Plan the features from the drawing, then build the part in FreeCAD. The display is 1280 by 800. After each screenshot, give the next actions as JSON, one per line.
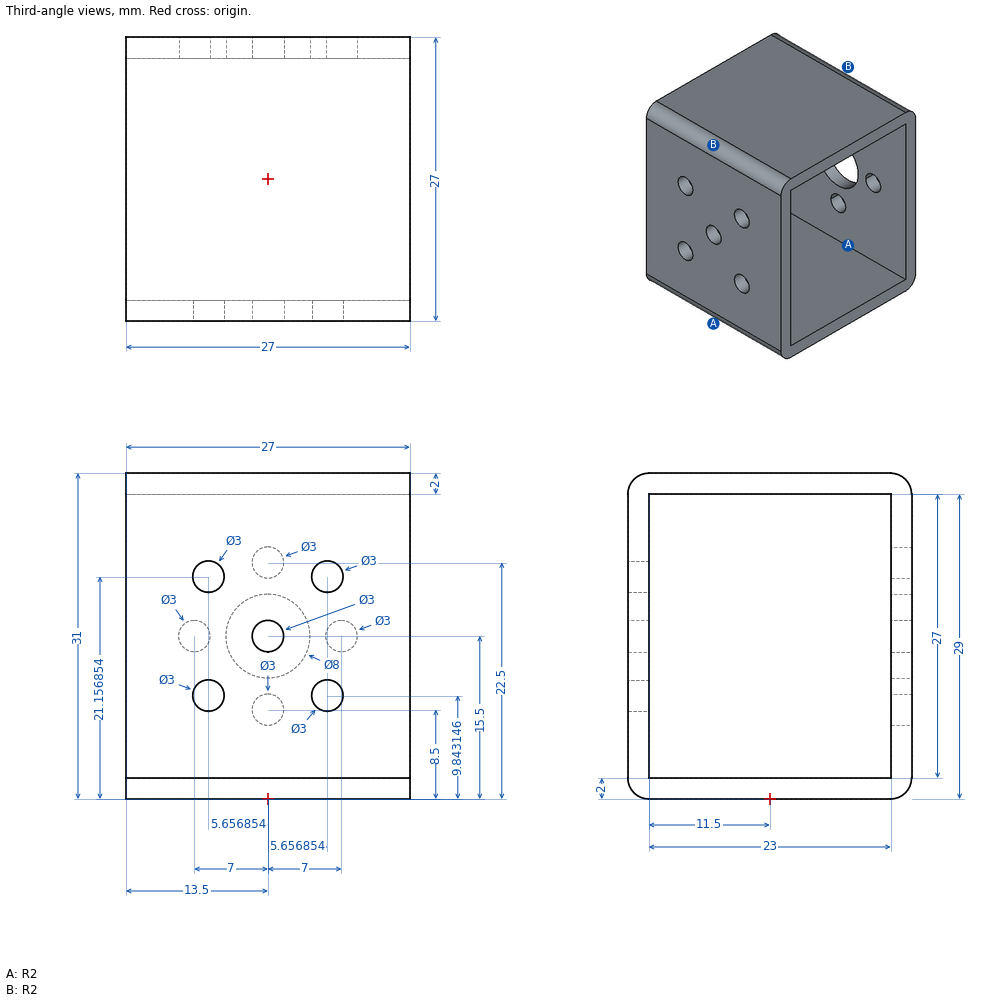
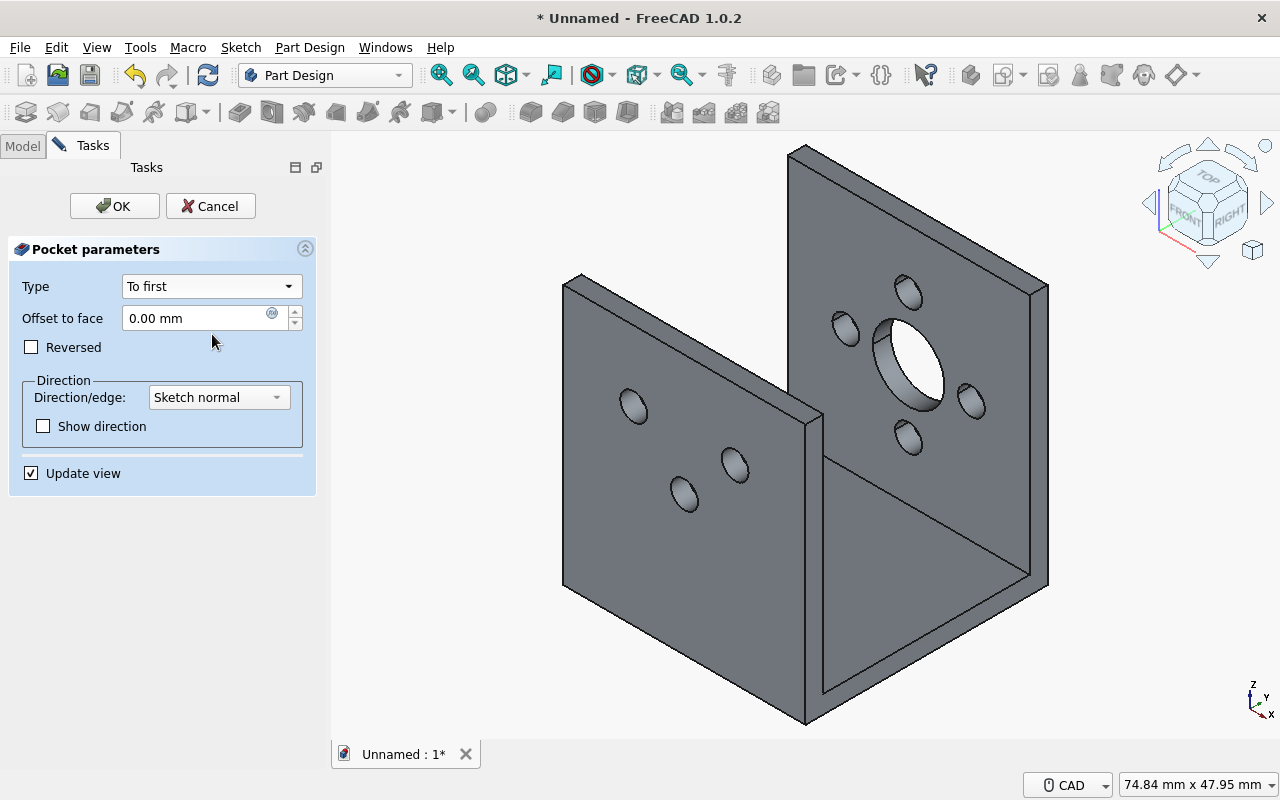
{"action": "left_click", "coordinate": [115, 206]}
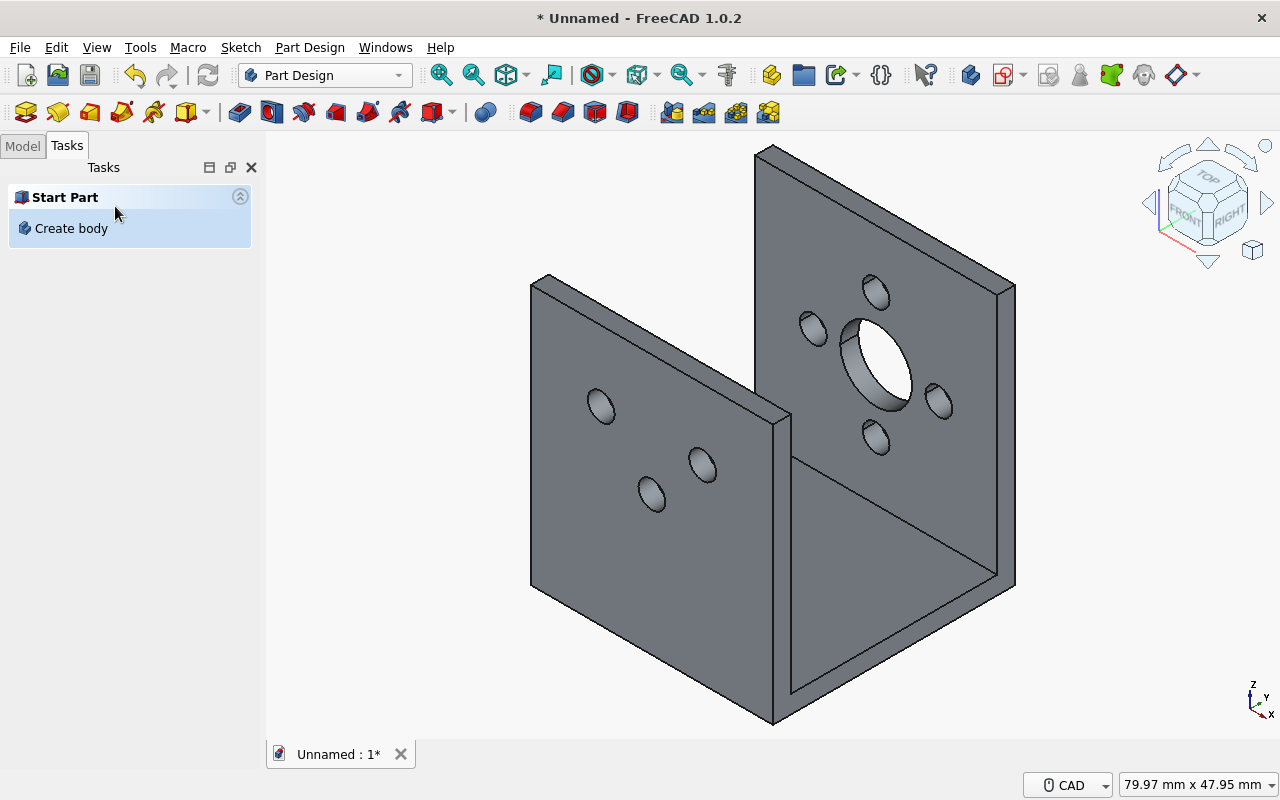
{"action": "left_click", "coordinate": [687, 610]}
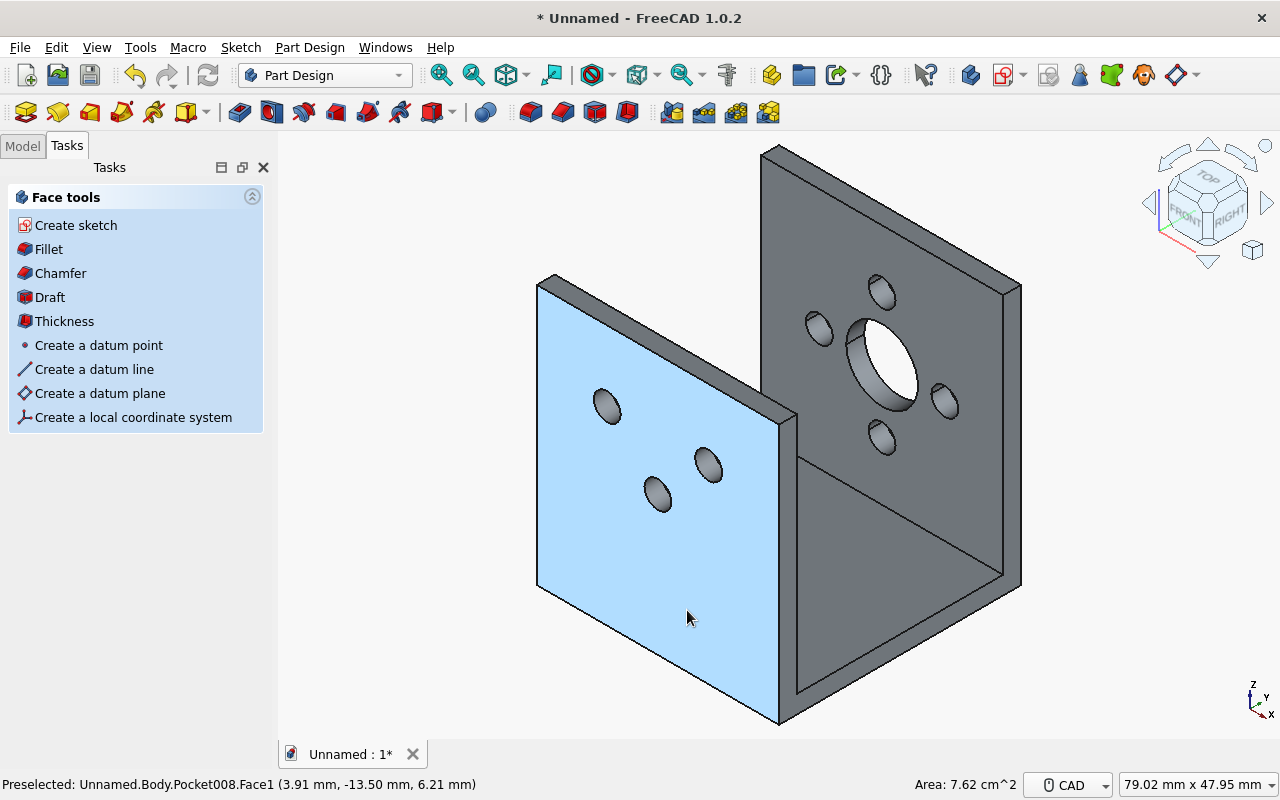
{"action": "left_click", "coordinate": [1004, 76]}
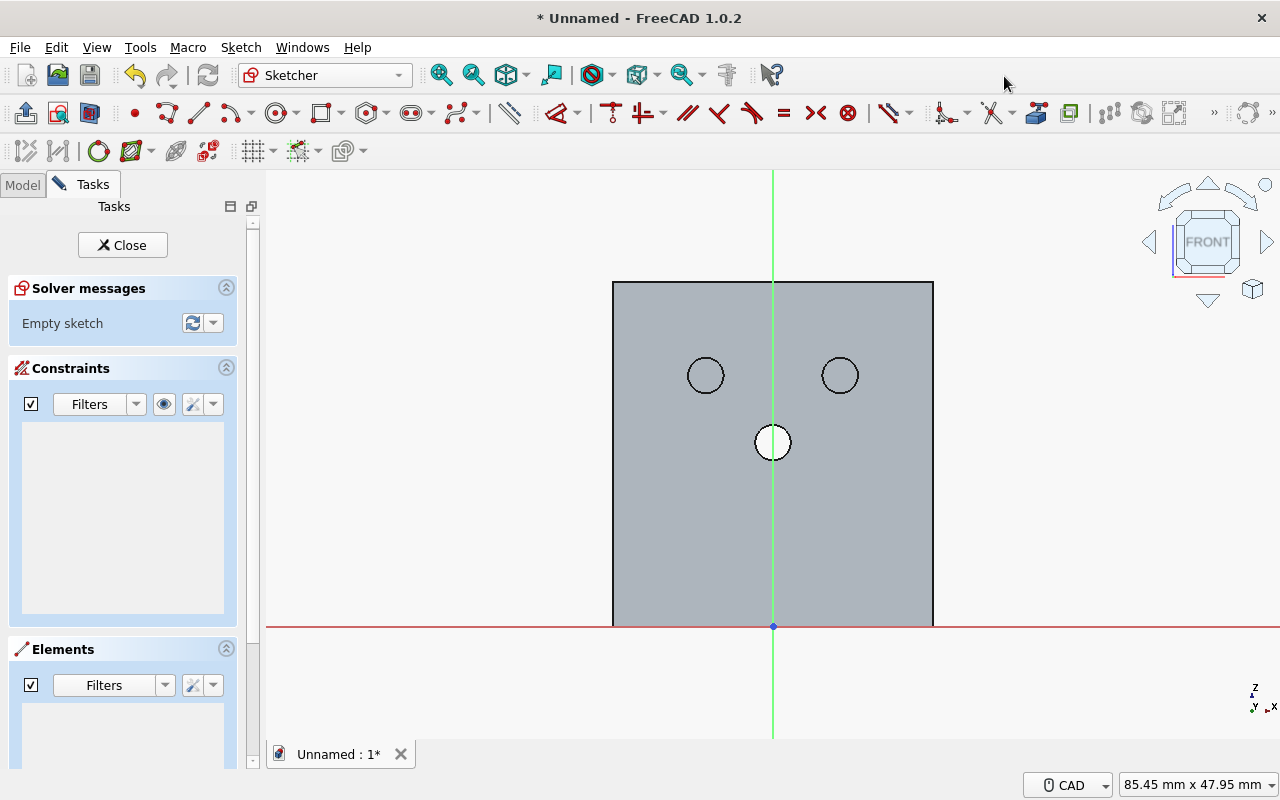
{"action": "scroll", "coordinate": [854, 515], "scroll_direction": "up", "scroll_amount": 12}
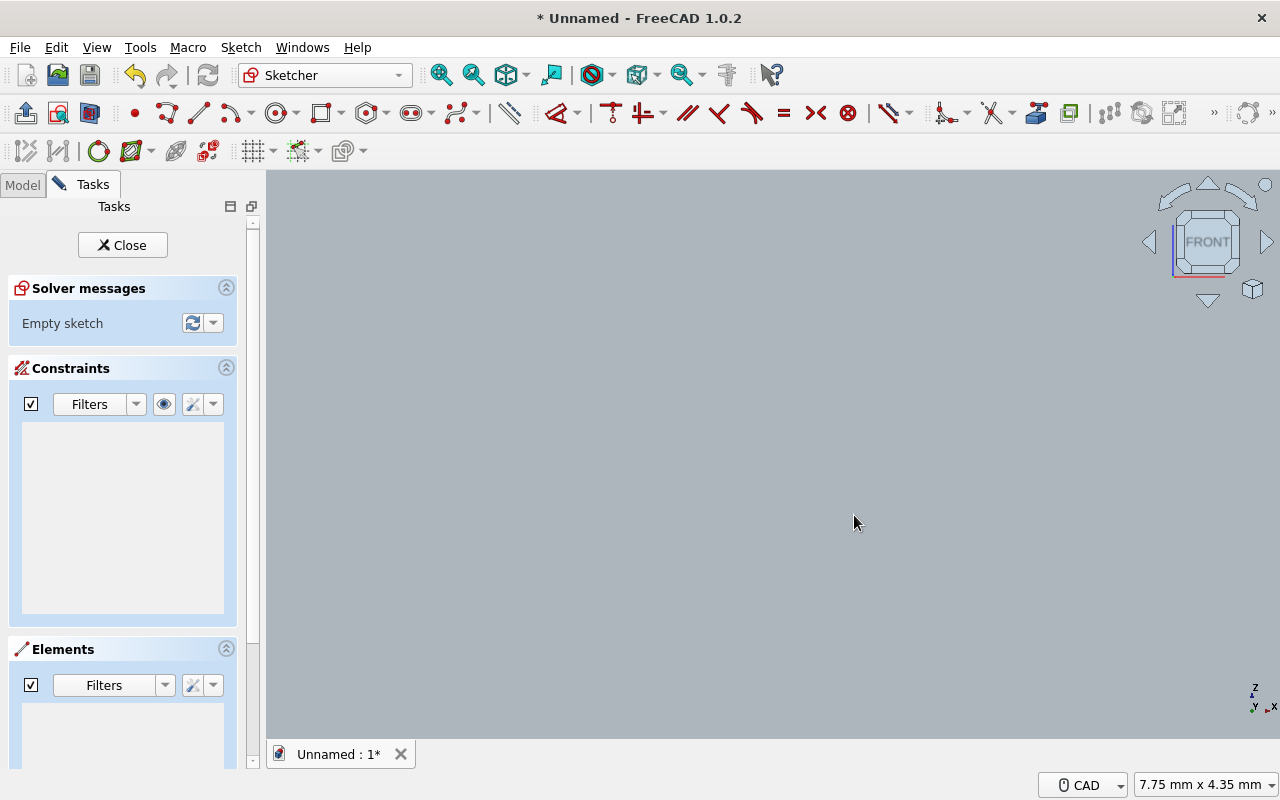
{"action": "left_click", "coordinate": [276, 114]}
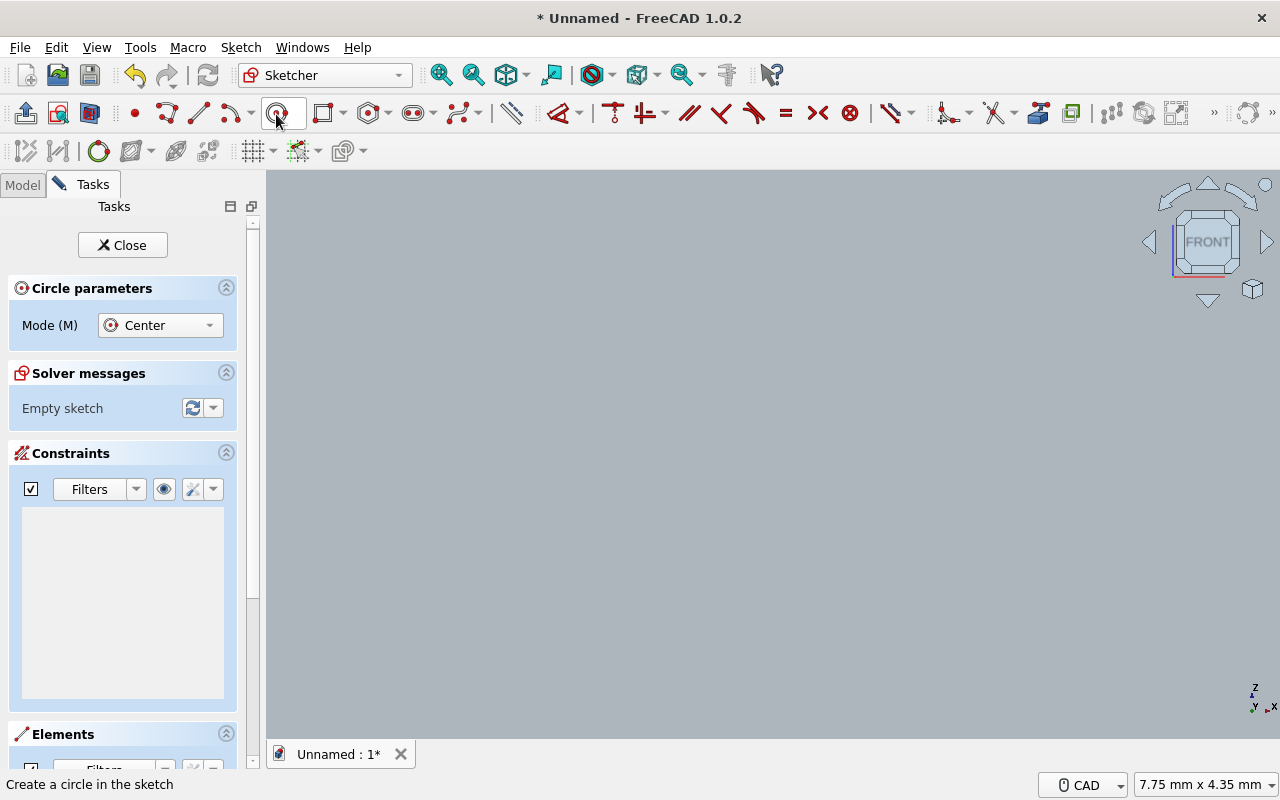
{"action": "left_click", "coordinate": [695, 451]}
{"action": "mouse_move", "coordinate": [834, 312]}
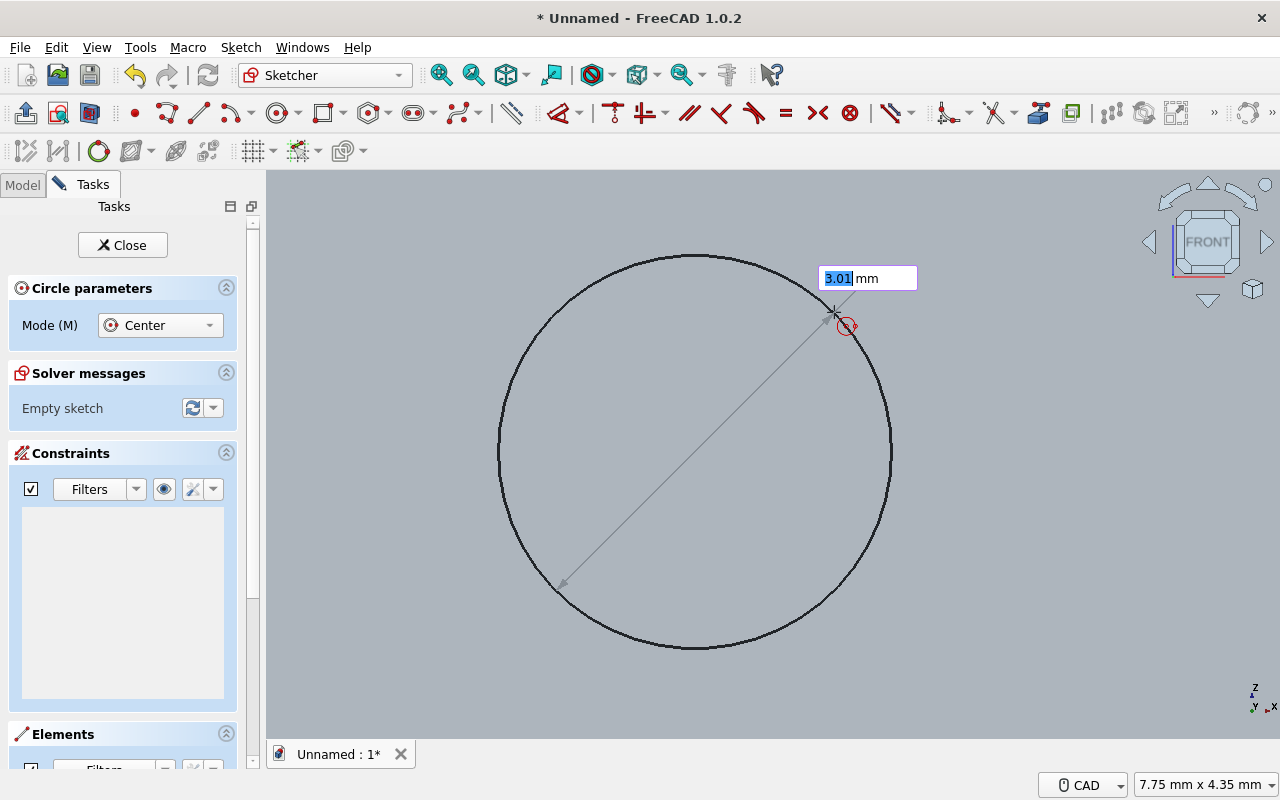
{"action": "type", "text": "3"}
{"action": "key", "text": "Return"}
{"action": "key", "text": "Escape"}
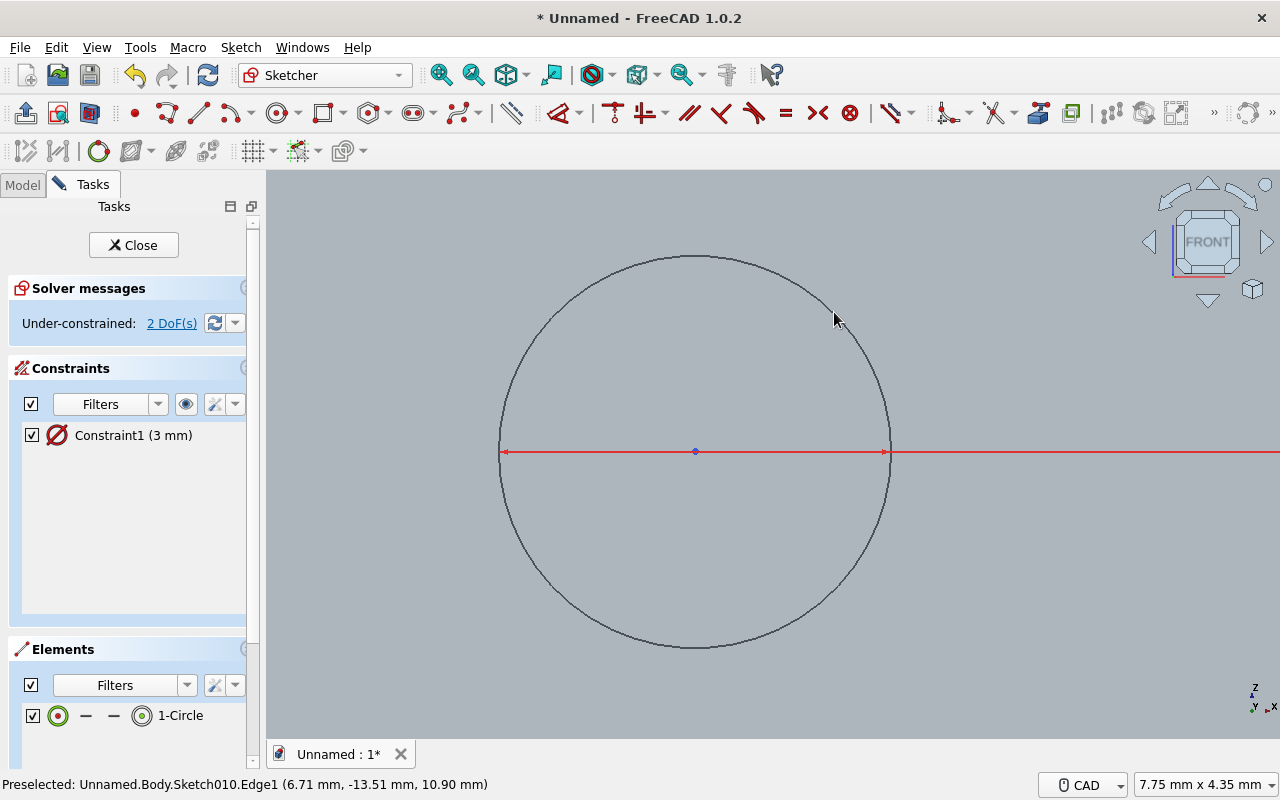
{"action": "left_click", "coordinate": [558, 114]}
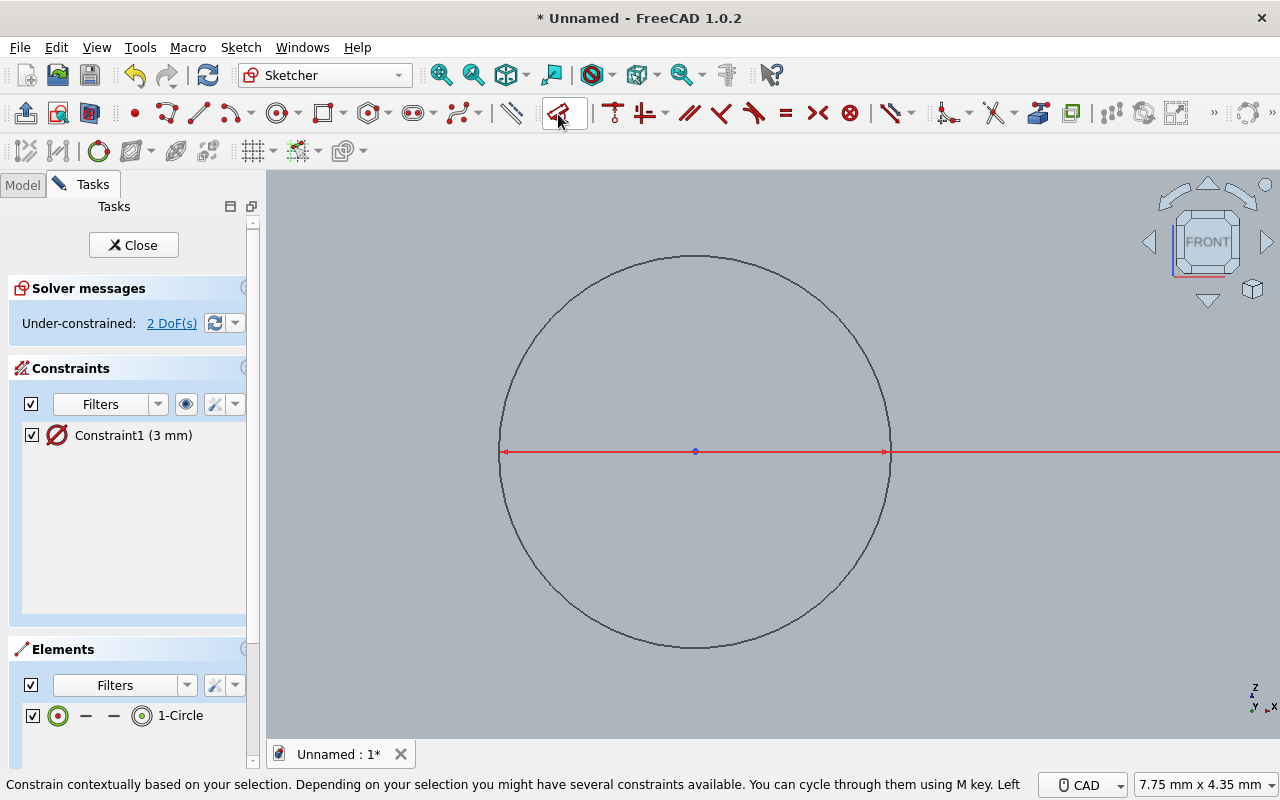
{"action": "left_click", "coordinate": [695, 452]}
{"action": "left_click", "coordinate": [402, 418]}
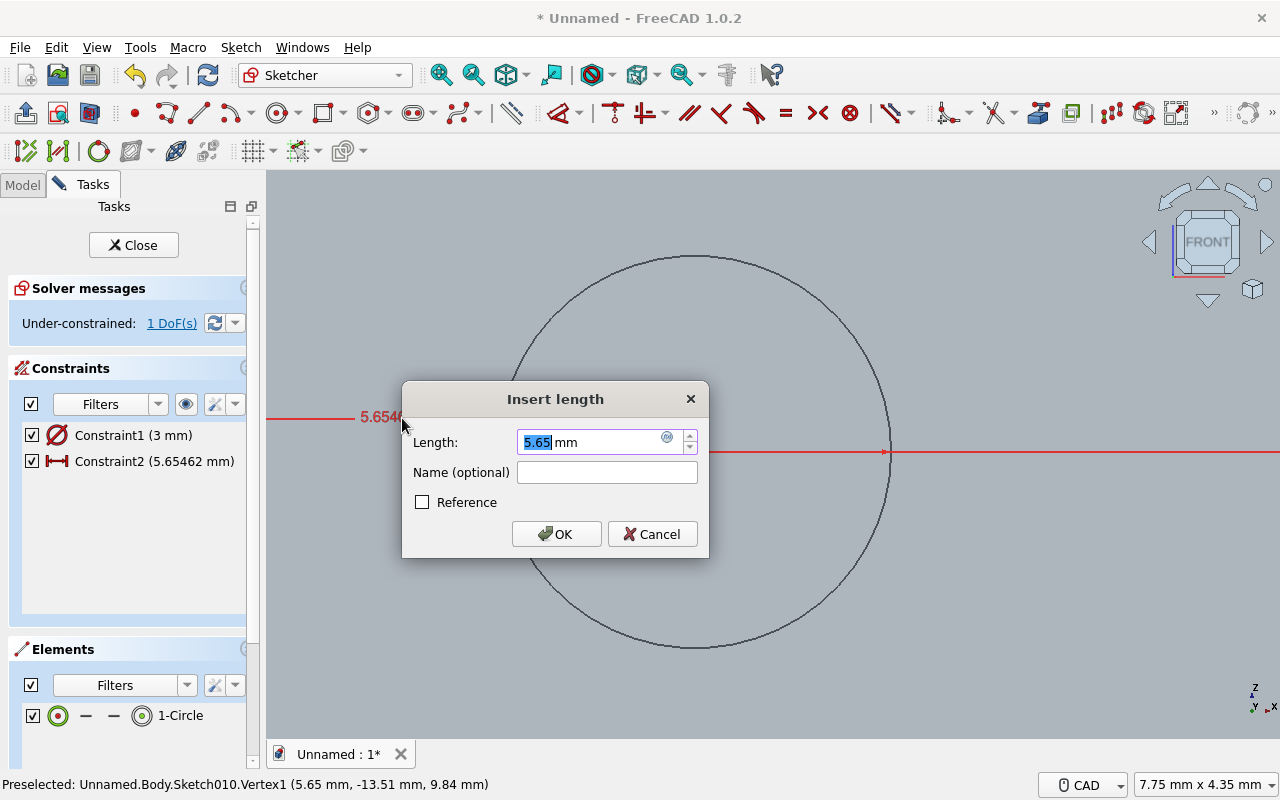
{"action": "type", "text": "5.656854"}
{"action": "key", "text": "Return"}